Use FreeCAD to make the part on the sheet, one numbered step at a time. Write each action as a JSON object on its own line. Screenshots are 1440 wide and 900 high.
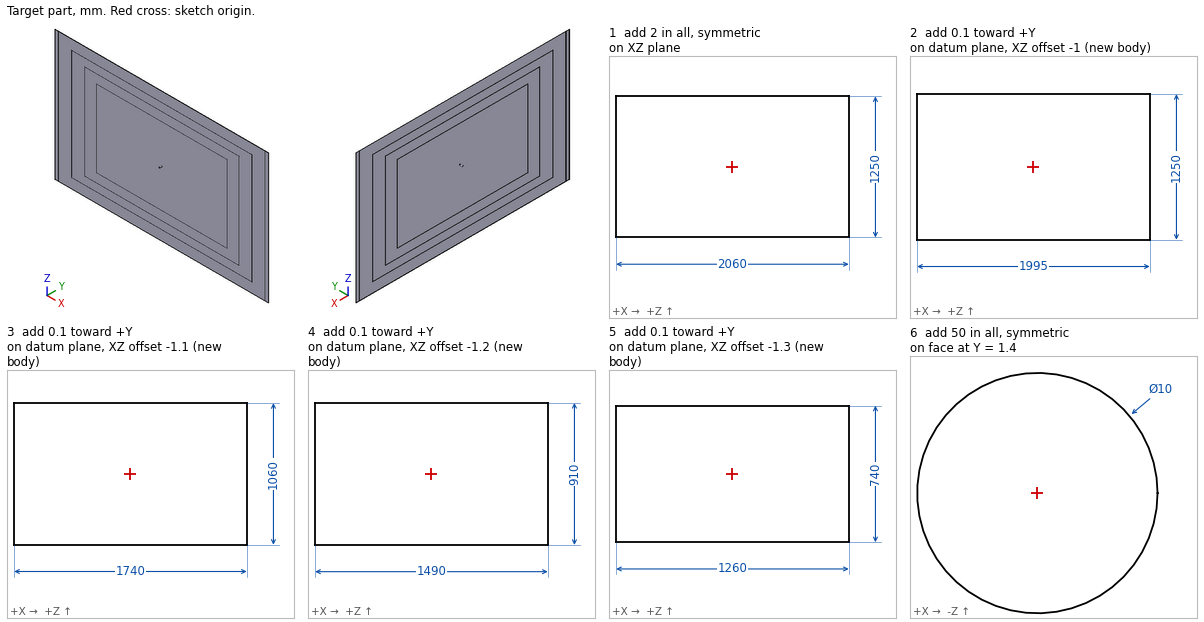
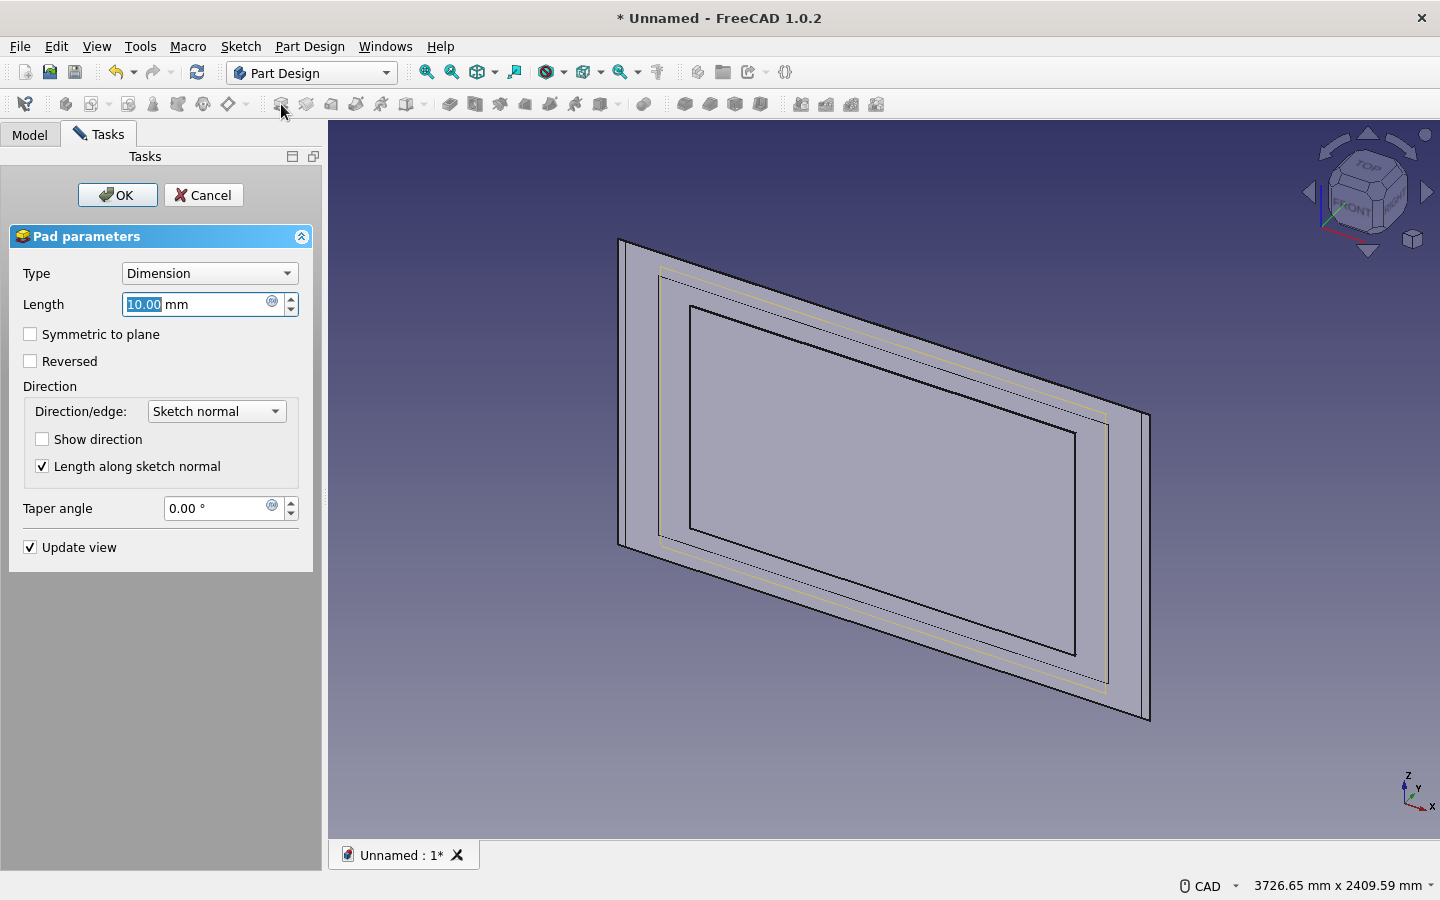
{"action": "type", "text": "0.1"}
{"action": "key", "text": "Tab"}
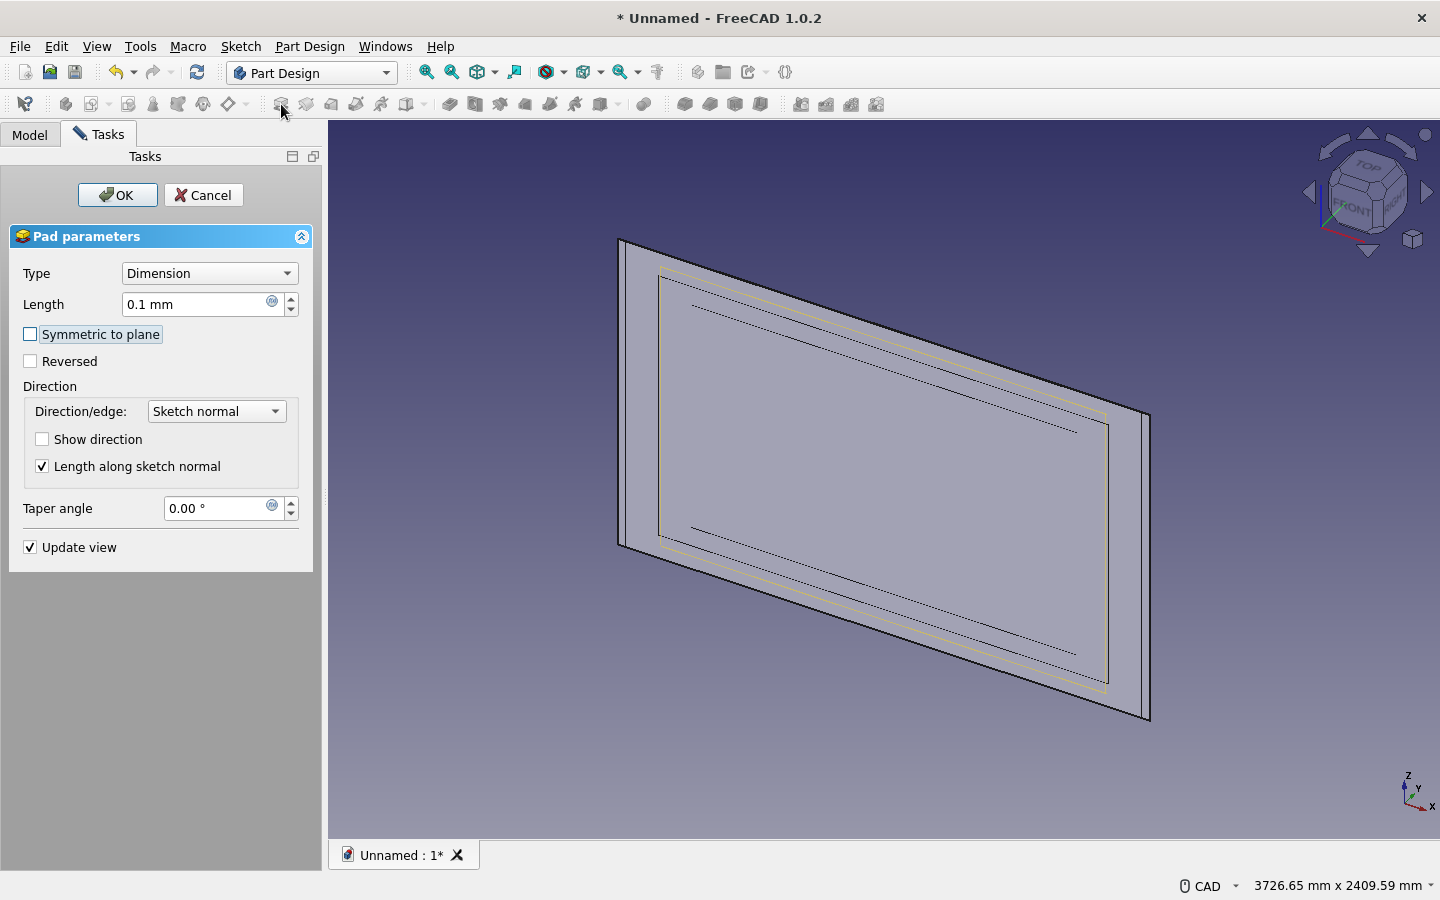
{"action": "left_click", "coordinate": [31, 361]}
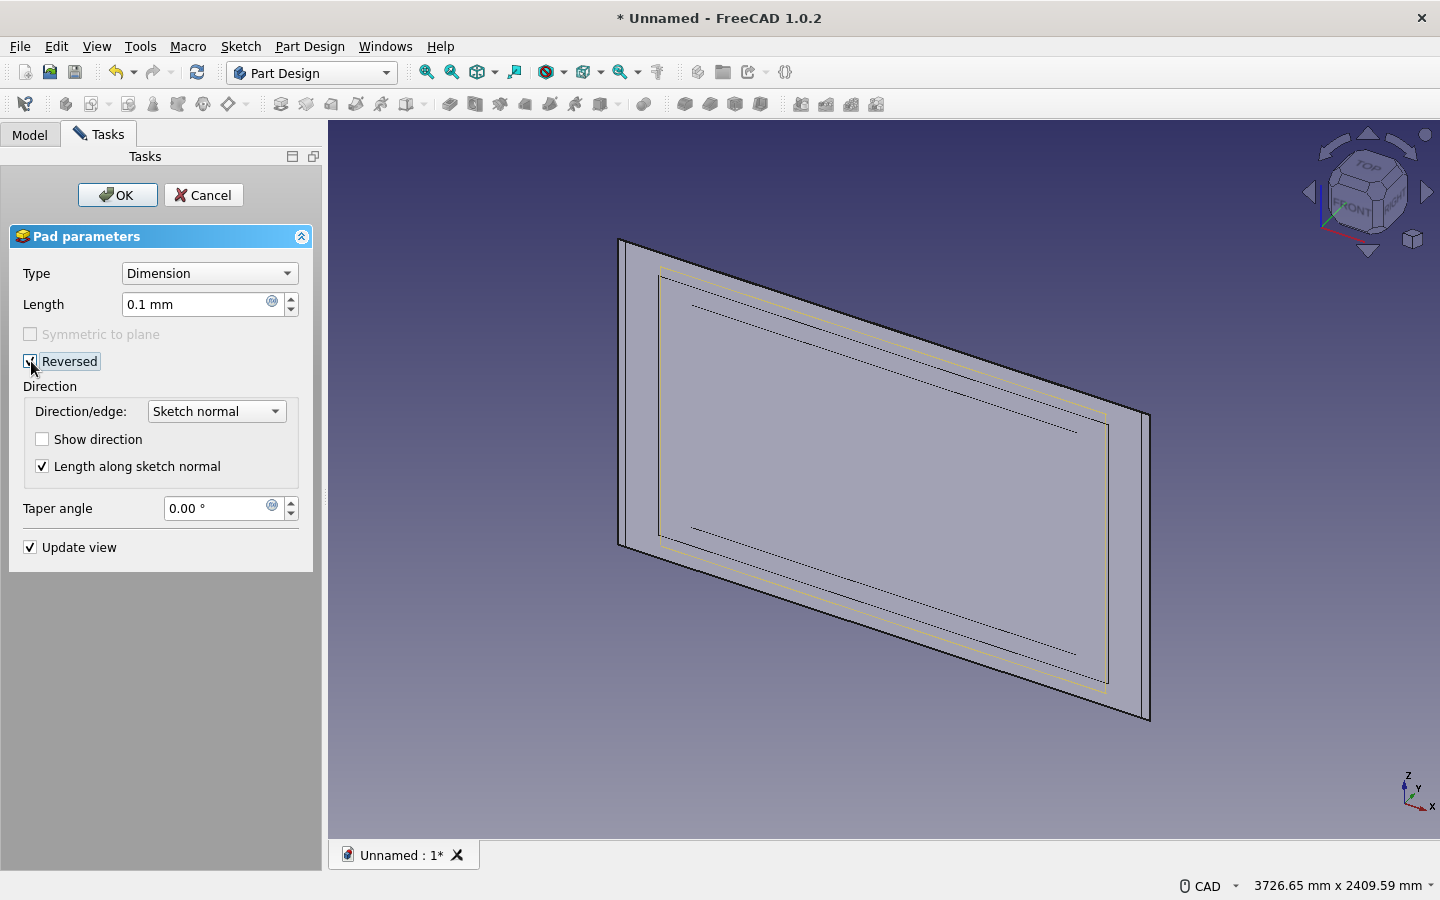
{"action": "left_click", "coordinate": [118, 195]}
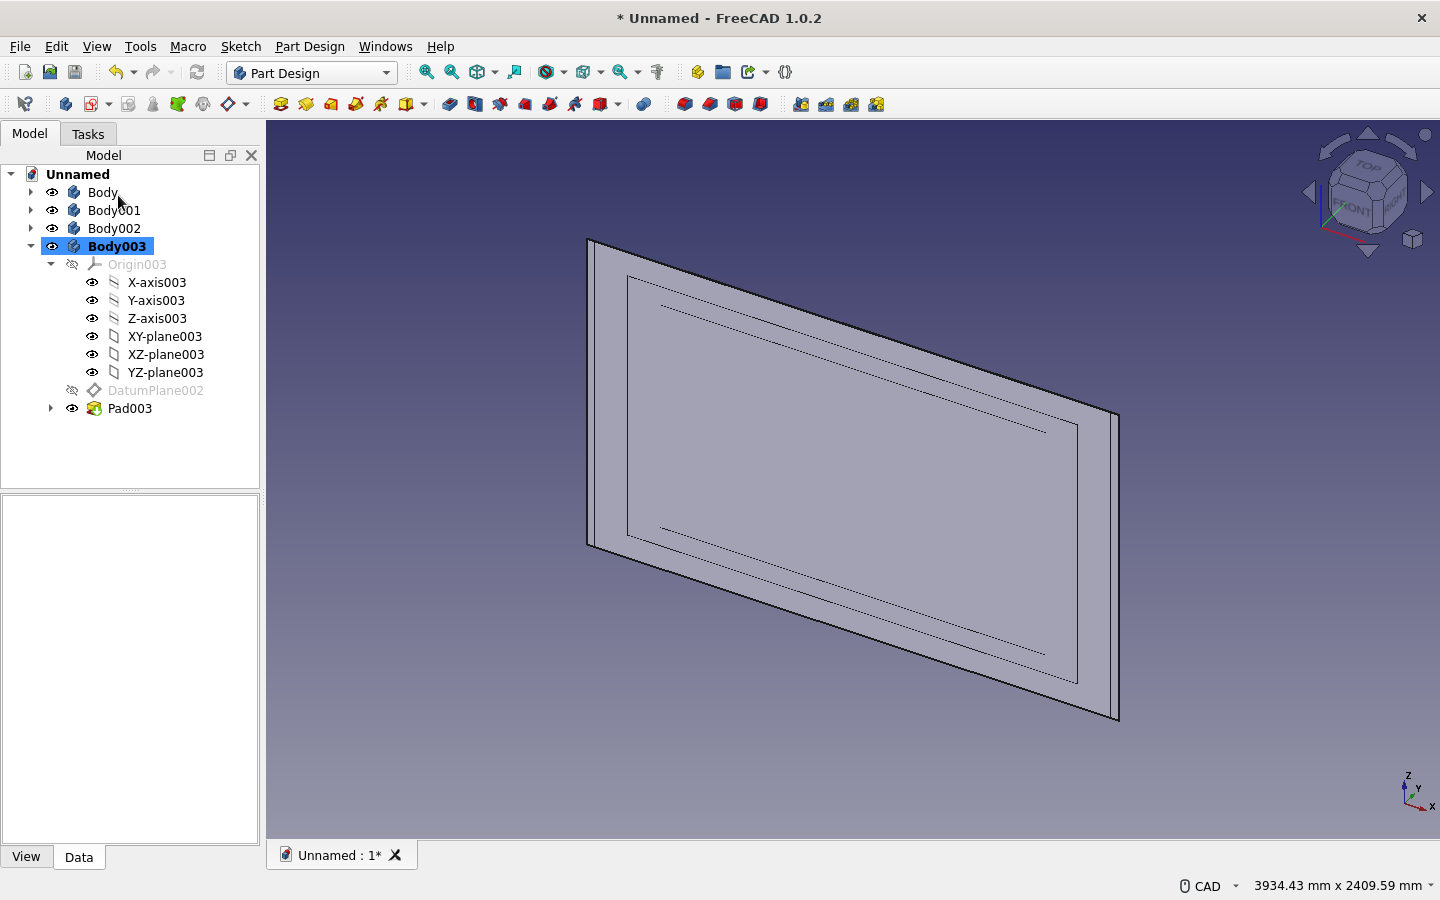
{"action": "left_click", "coordinate": [66, 104]}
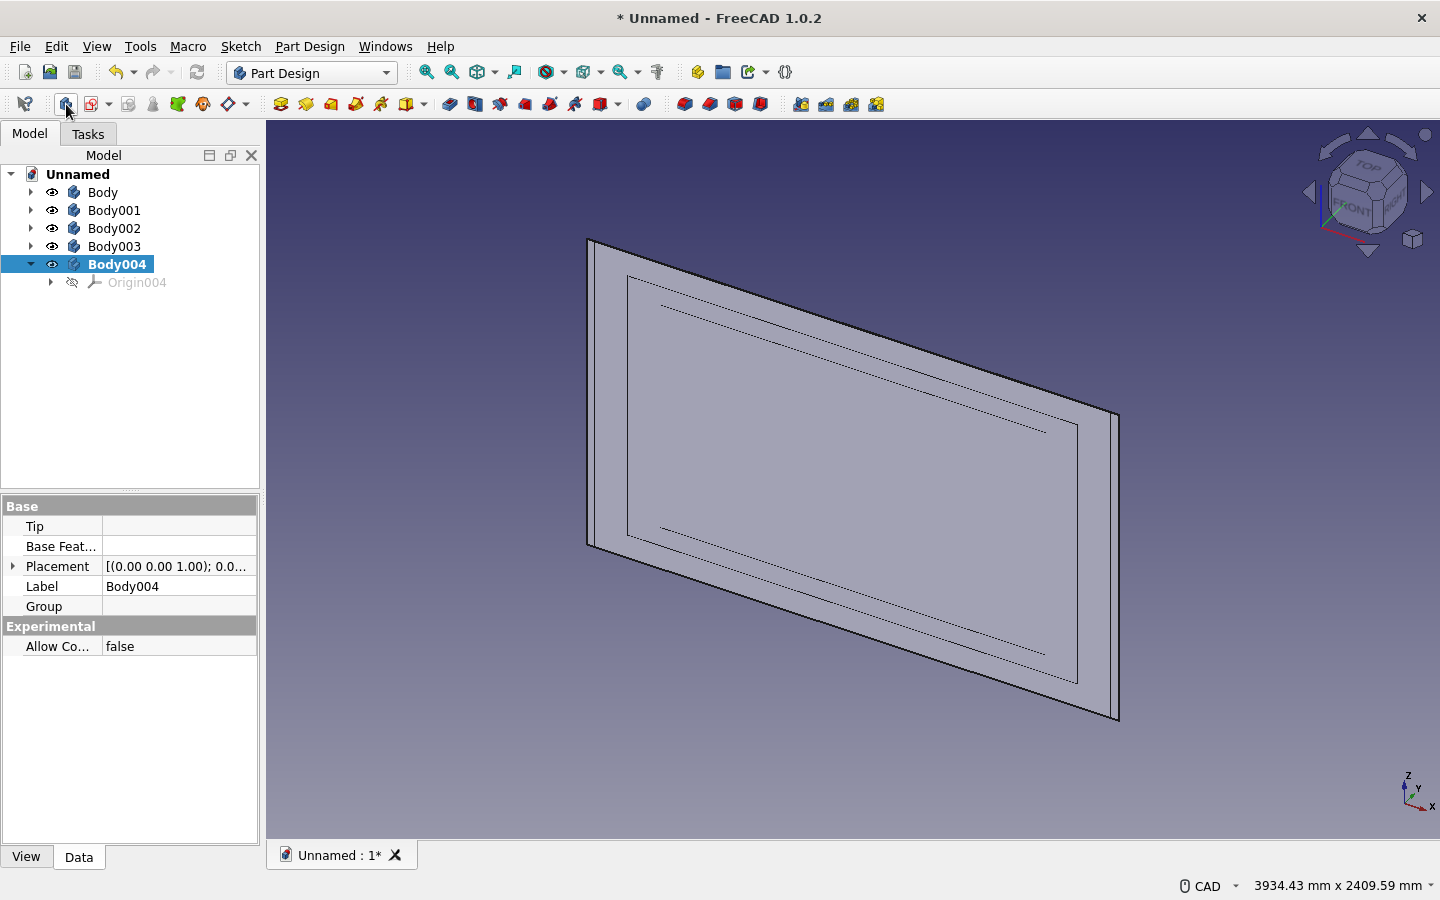
{"action": "left_click", "coordinate": [51, 282]}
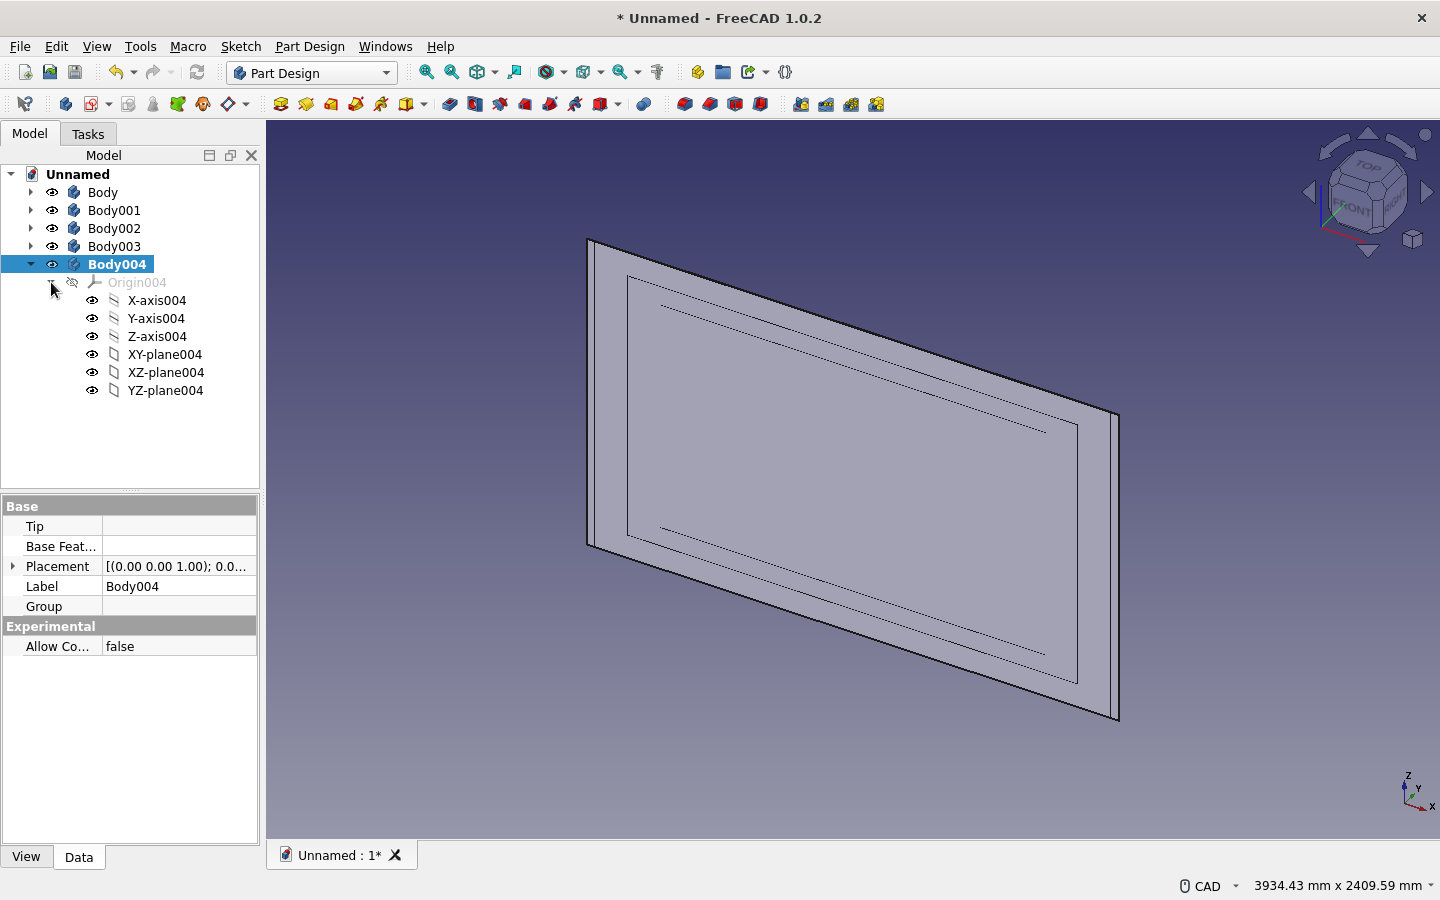
{"action": "left_click", "coordinate": [137, 372]}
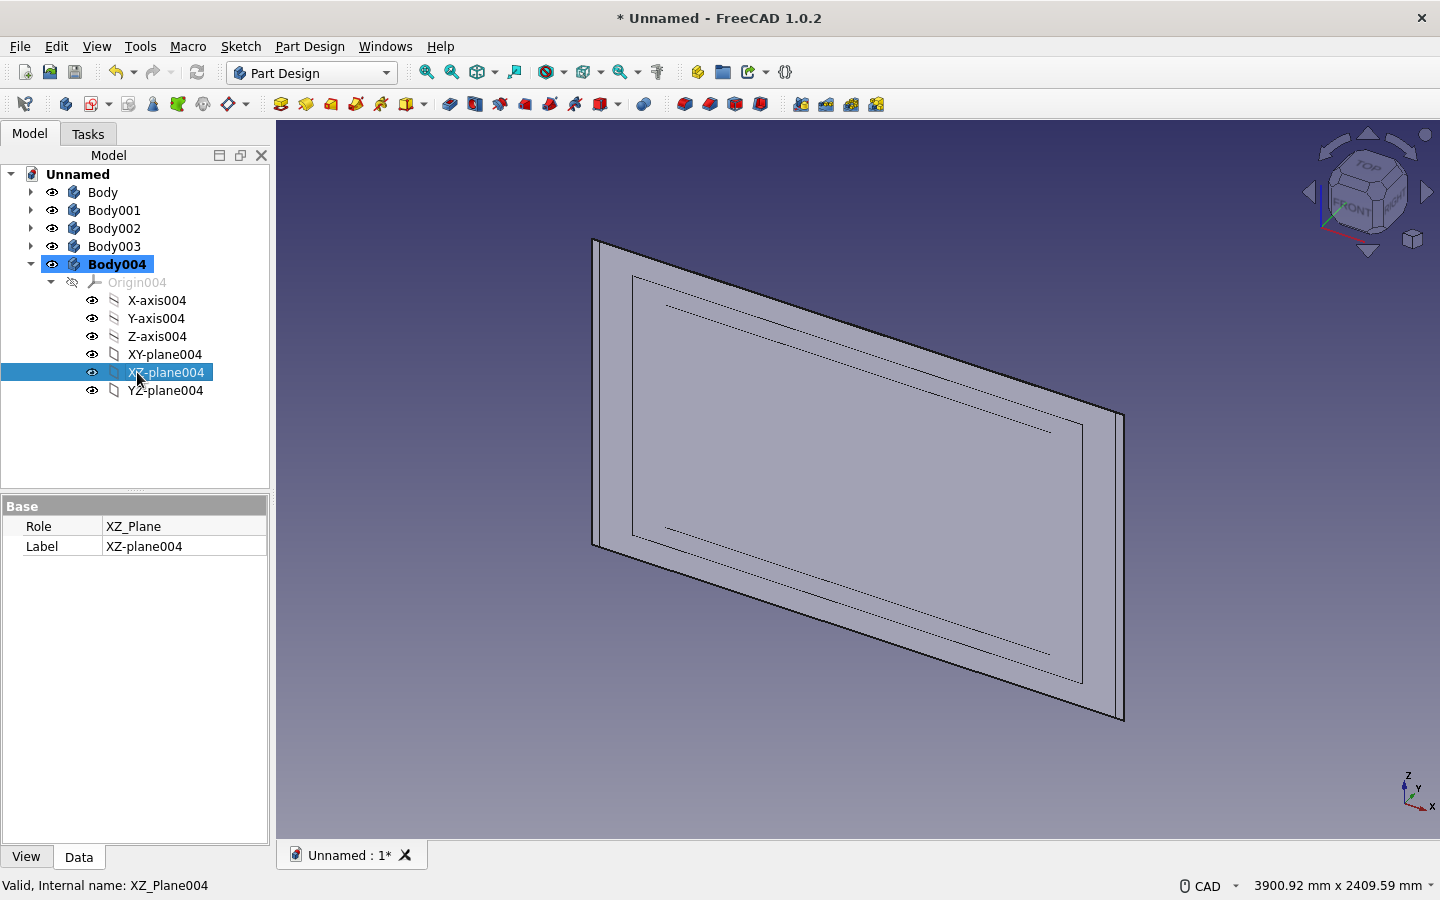
{"action": "left_click", "coordinate": [228, 104]}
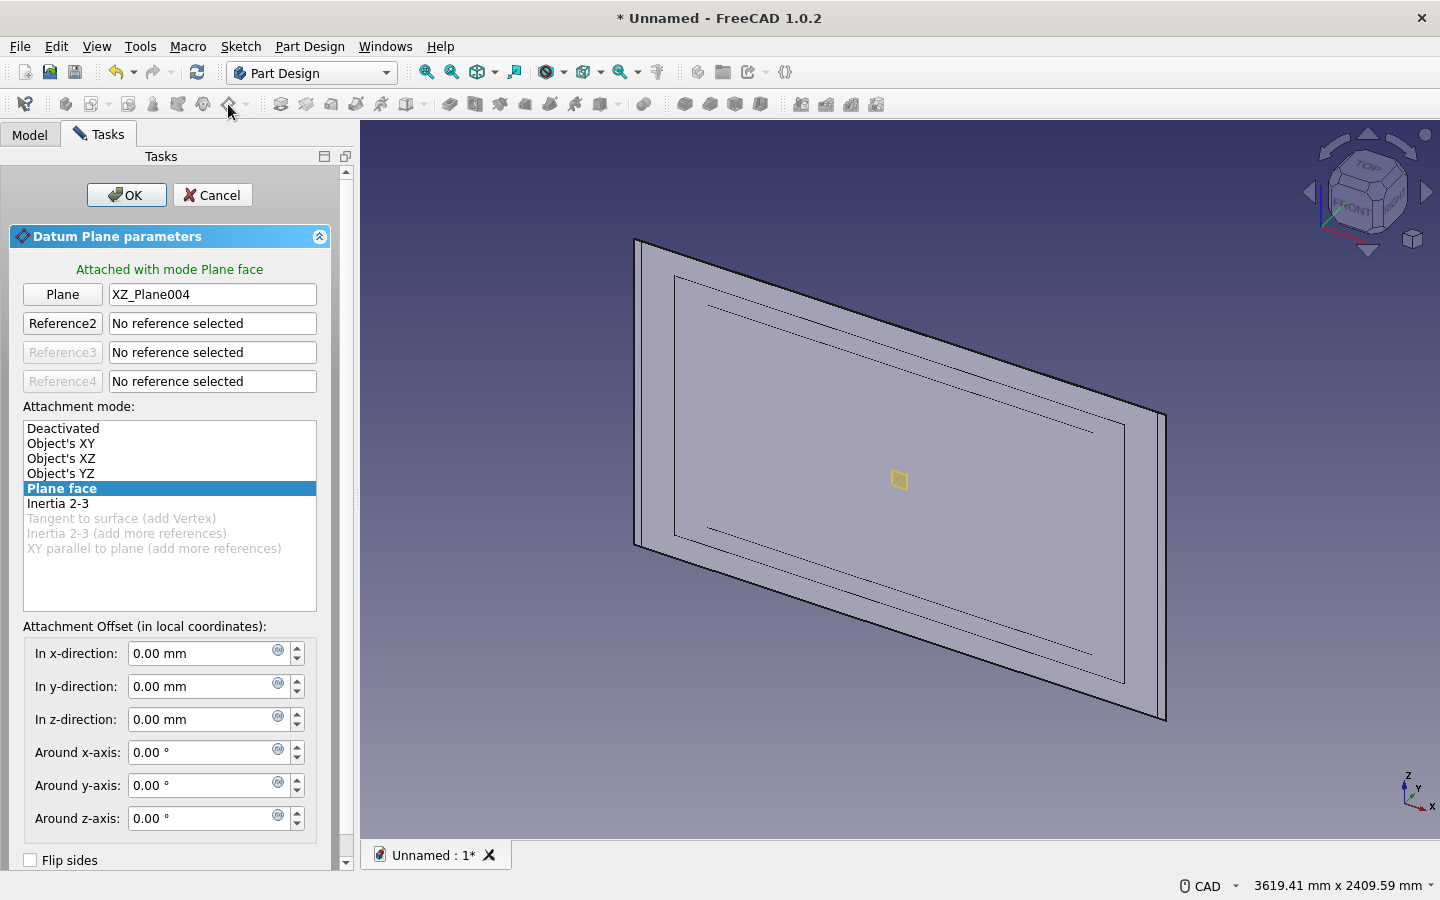
{"action": "triple_click", "coordinate": [210, 720]}